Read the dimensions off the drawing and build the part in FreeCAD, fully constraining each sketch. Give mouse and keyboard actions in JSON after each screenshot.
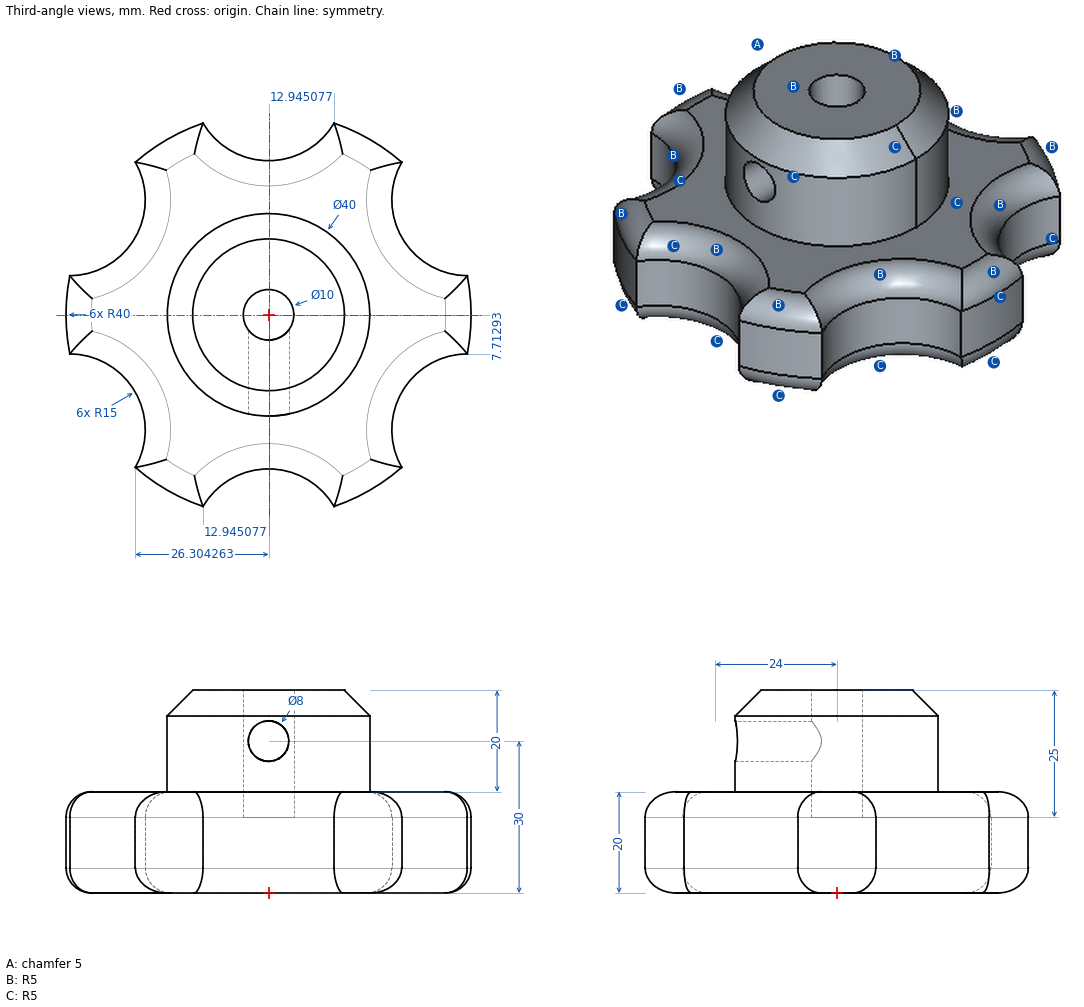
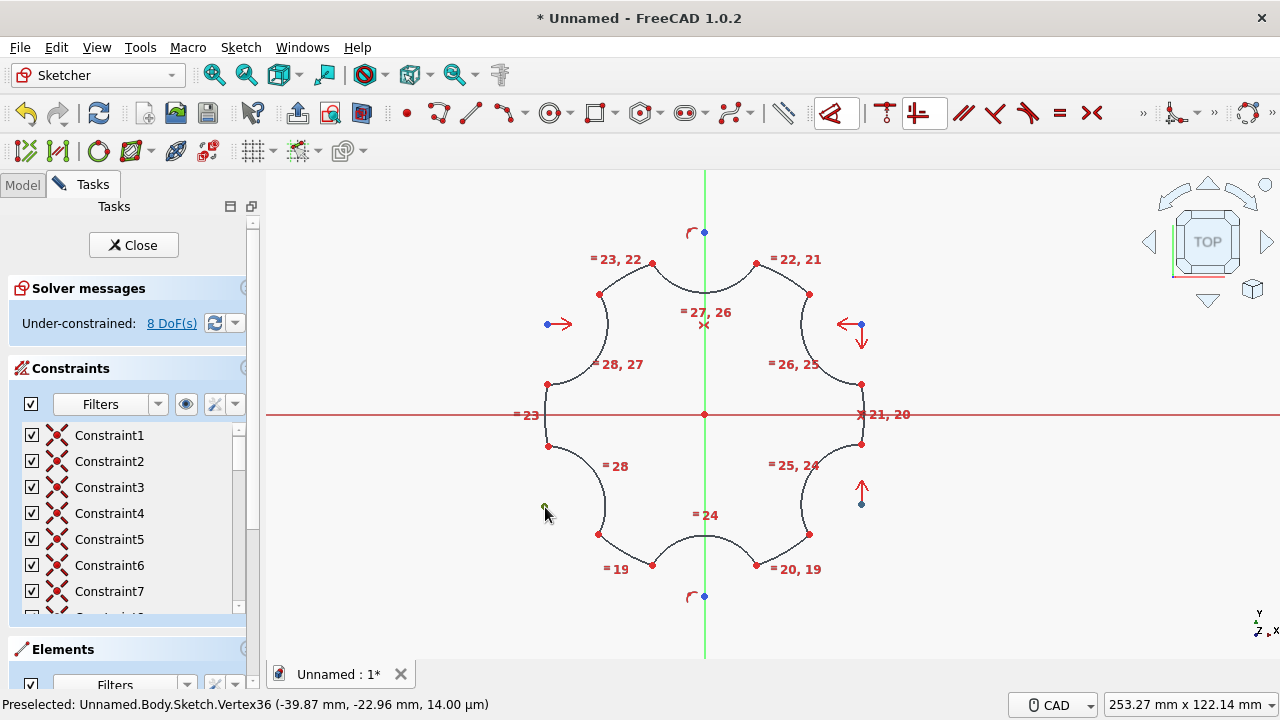
{"action": "left_click", "coordinate": [705, 569]}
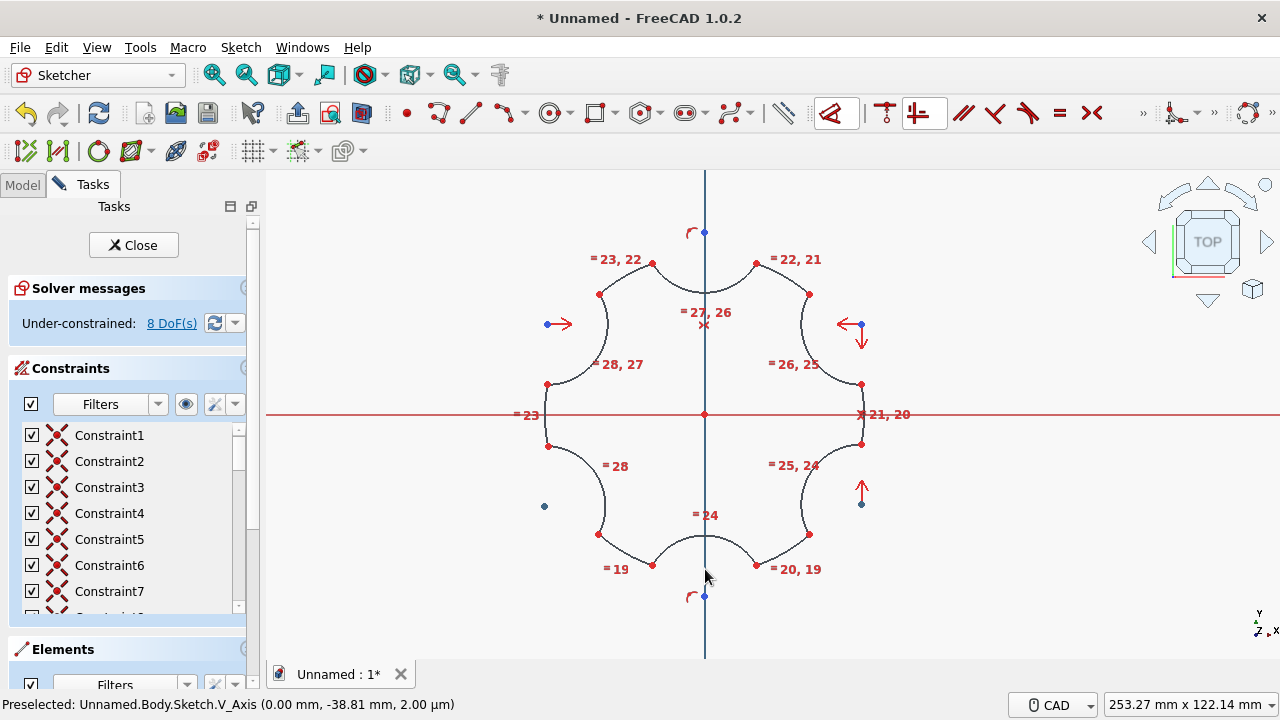
{"action": "left_click", "coordinate": [1092, 114]}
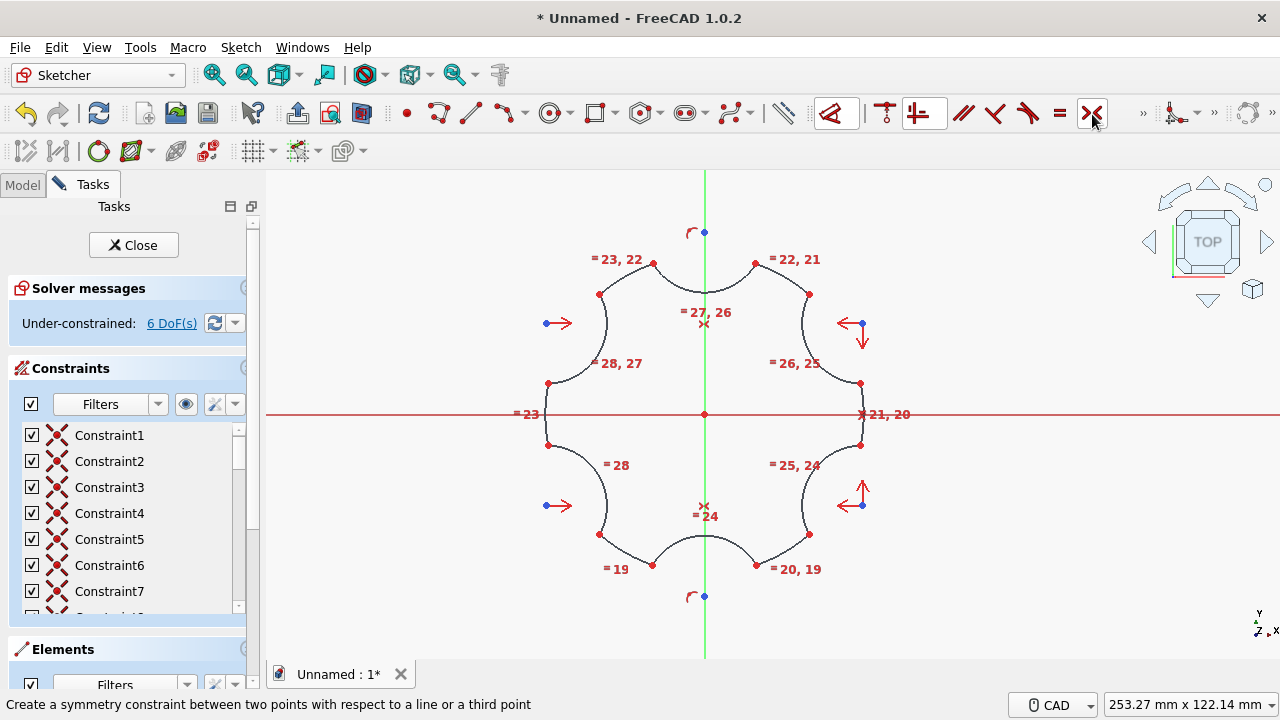
{"action": "left_click", "coordinate": [830, 114]}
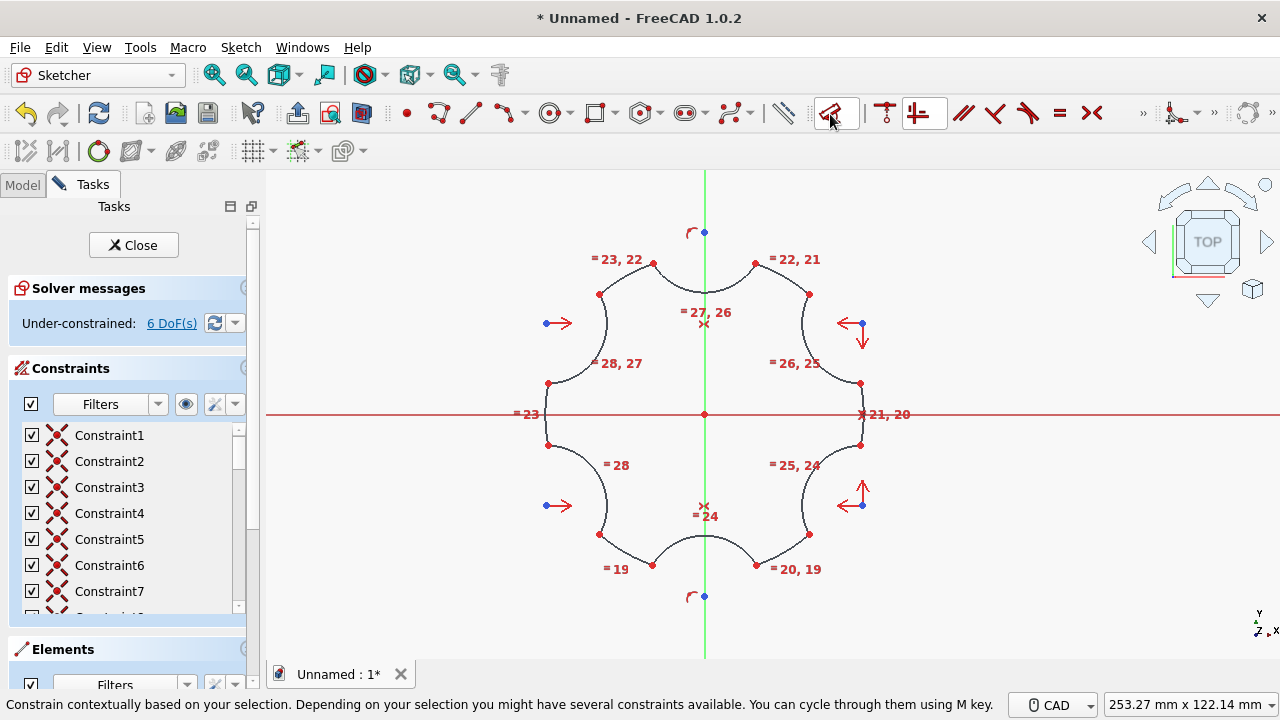
{"action": "left_click", "coordinate": [614, 546]}
{"action": "left_click", "coordinate": [596, 572]}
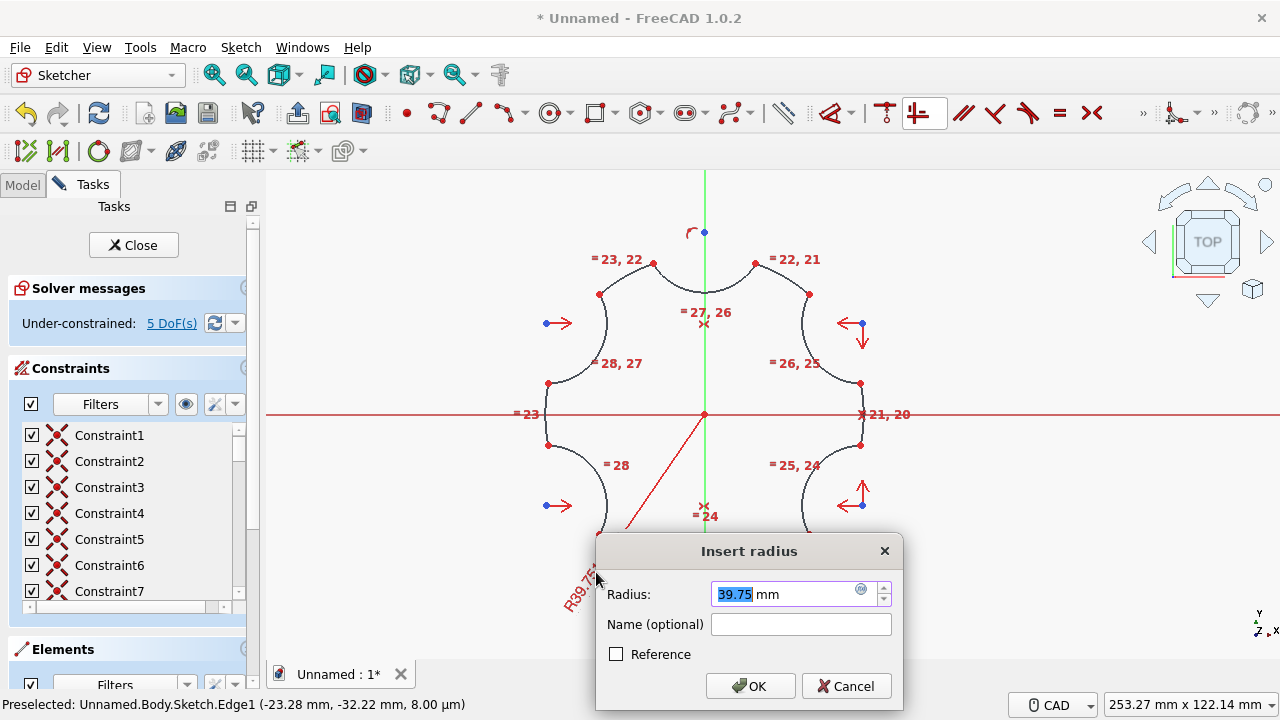
{"action": "type", "text": "40"}
{"action": "key", "text": "Return"}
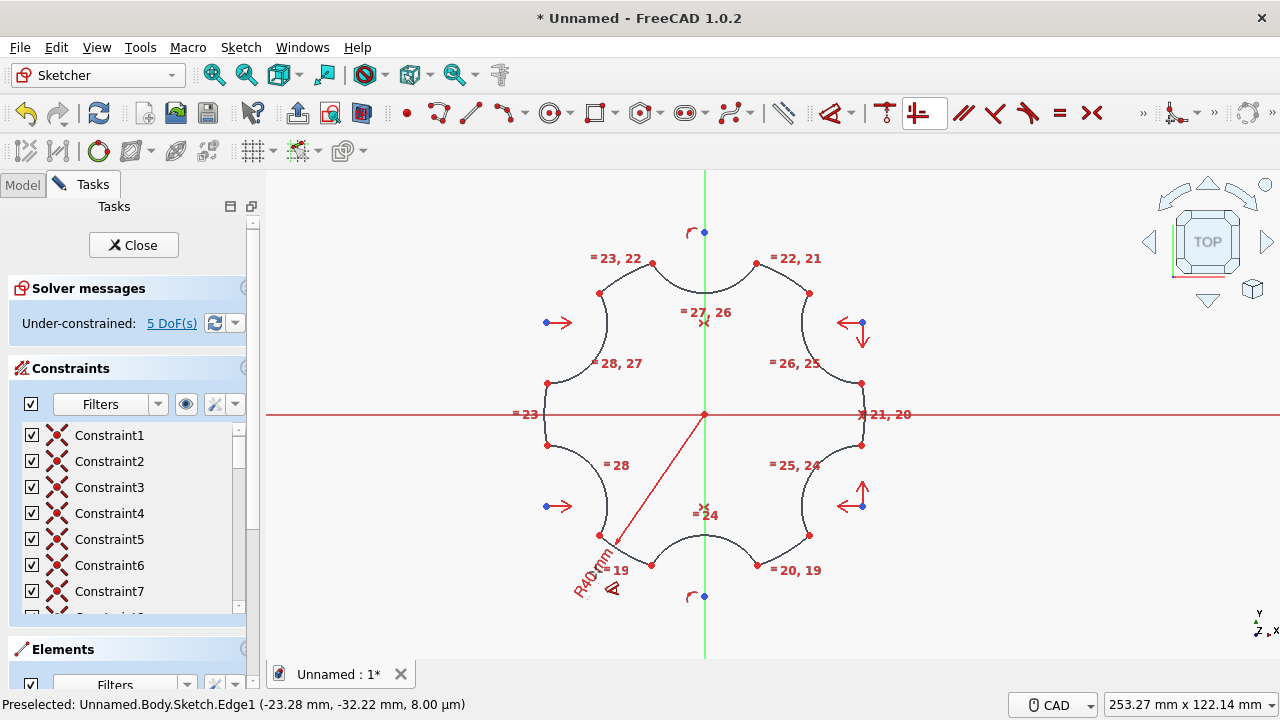
{"action": "left_click", "coordinate": [729, 541]}
{"action": "left_click", "coordinate": [742, 512]}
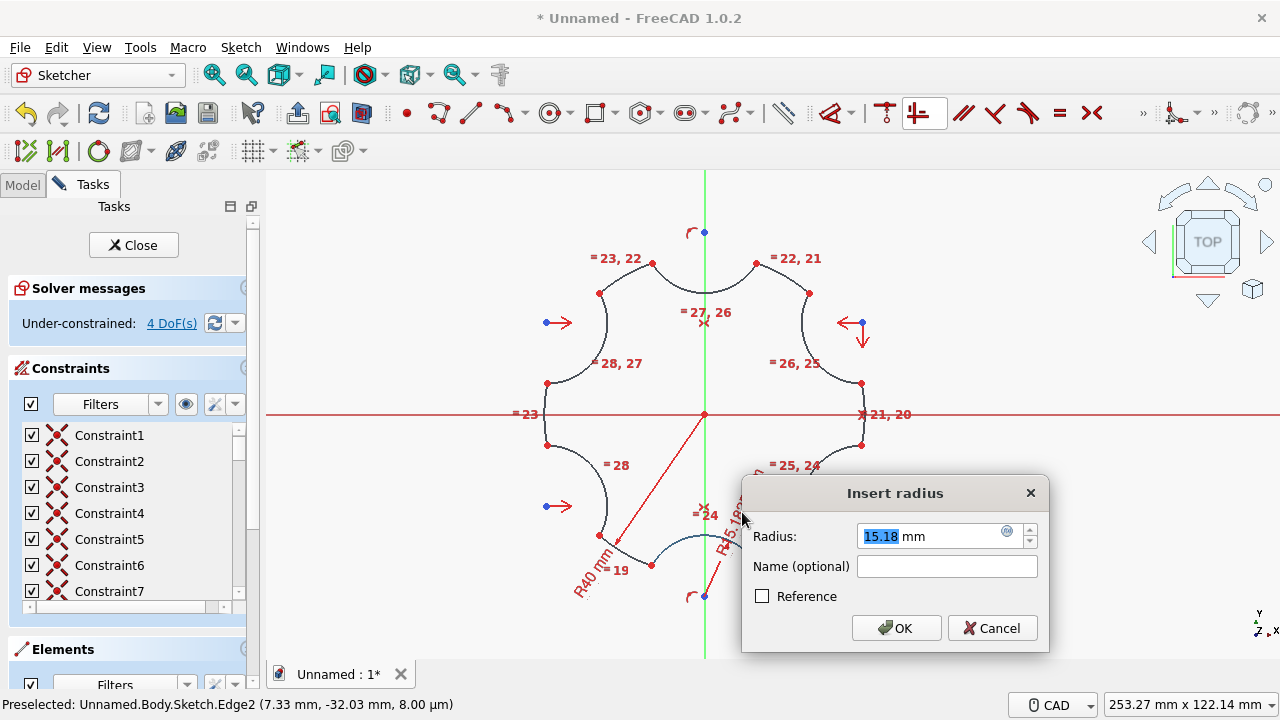
{"action": "type", "text": "15"}
{"action": "key", "text": "Return"}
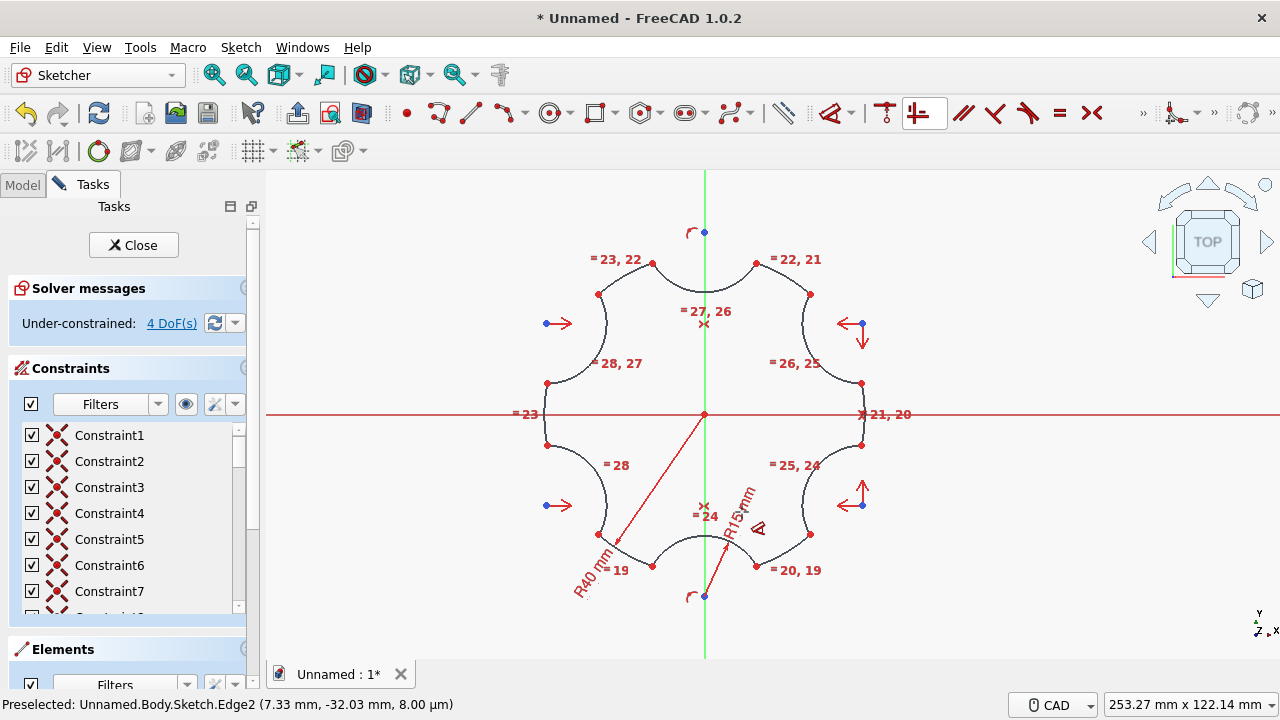
{"action": "scroll", "coordinate": [862, 446], "scroll_direction": "up", "scroll_amount": 2}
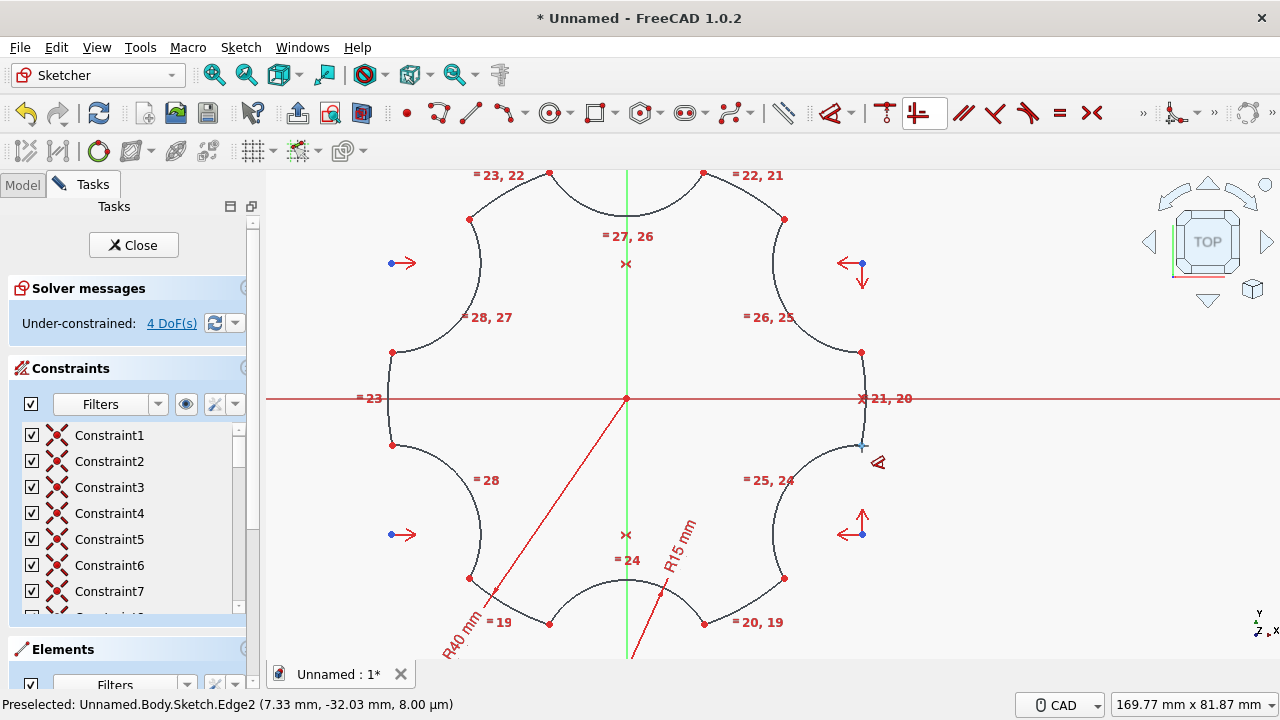
{"action": "left_click", "coordinate": [861, 445]}
{"action": "left_click", "coordinate": [895, 422]}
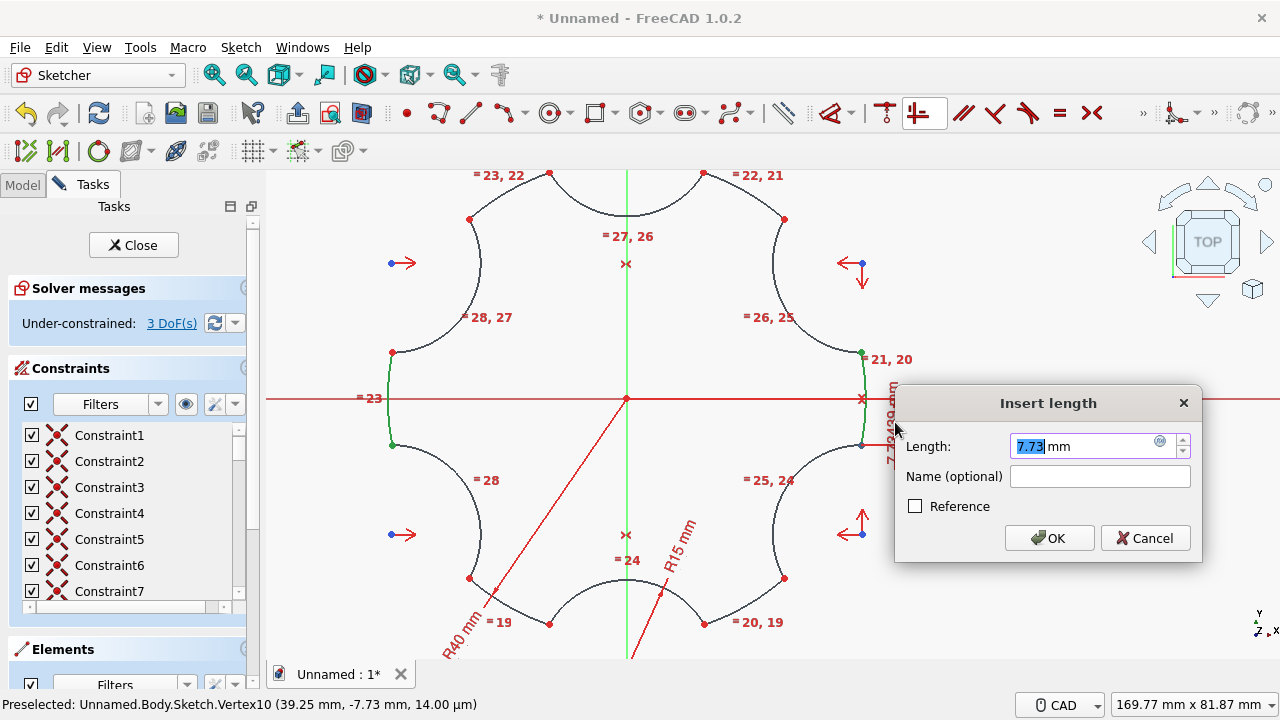
{"action": "type", "text": "7.71293"}
{"action": "key", "text": "Return"}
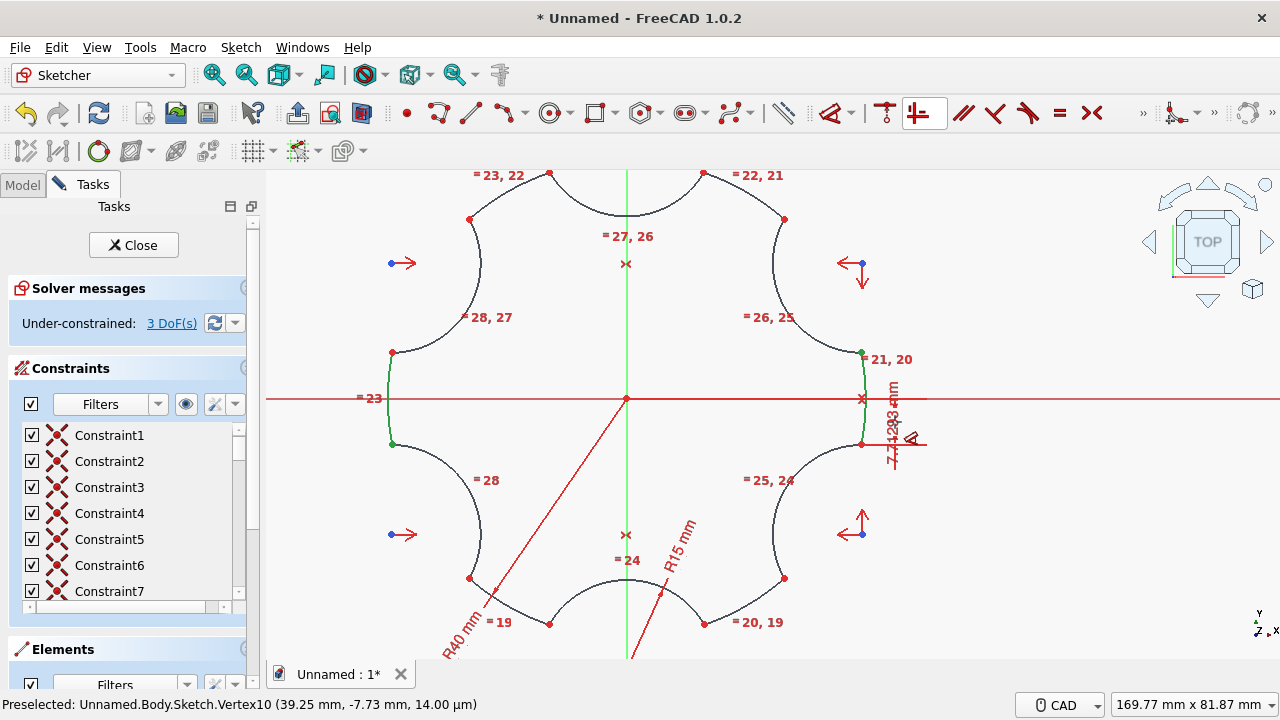
{"action": "left_click", "coordinate": [469, 578]}
{"action": "left_click", "coordinate": [584, 612]}